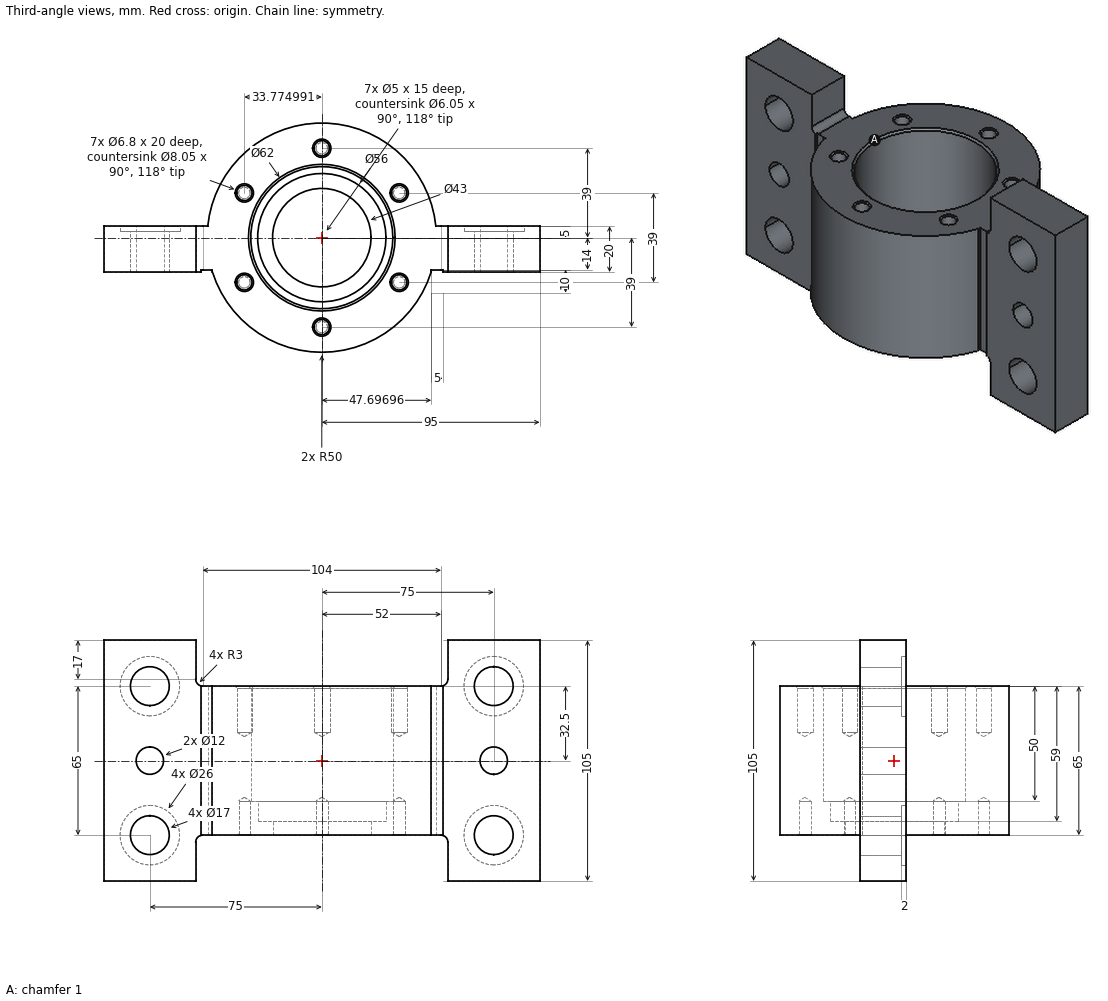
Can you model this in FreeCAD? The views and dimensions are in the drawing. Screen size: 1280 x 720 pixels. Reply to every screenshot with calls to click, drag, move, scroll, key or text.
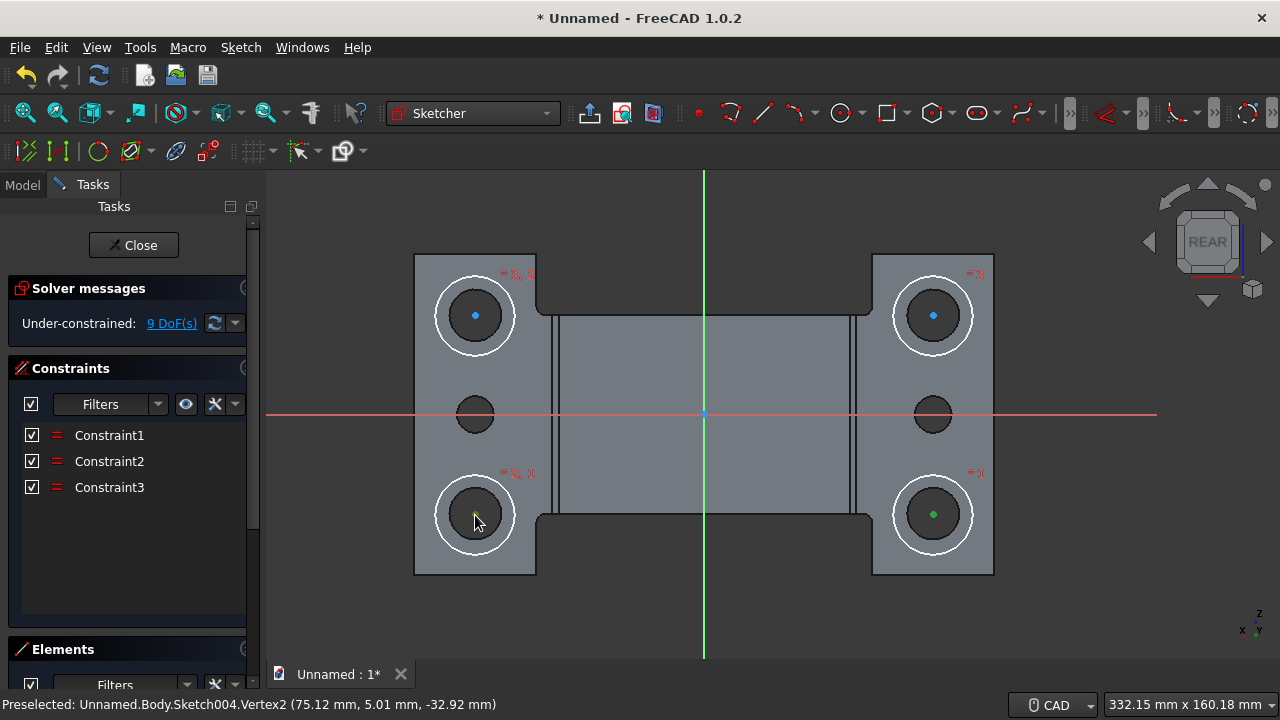
click(704, 600)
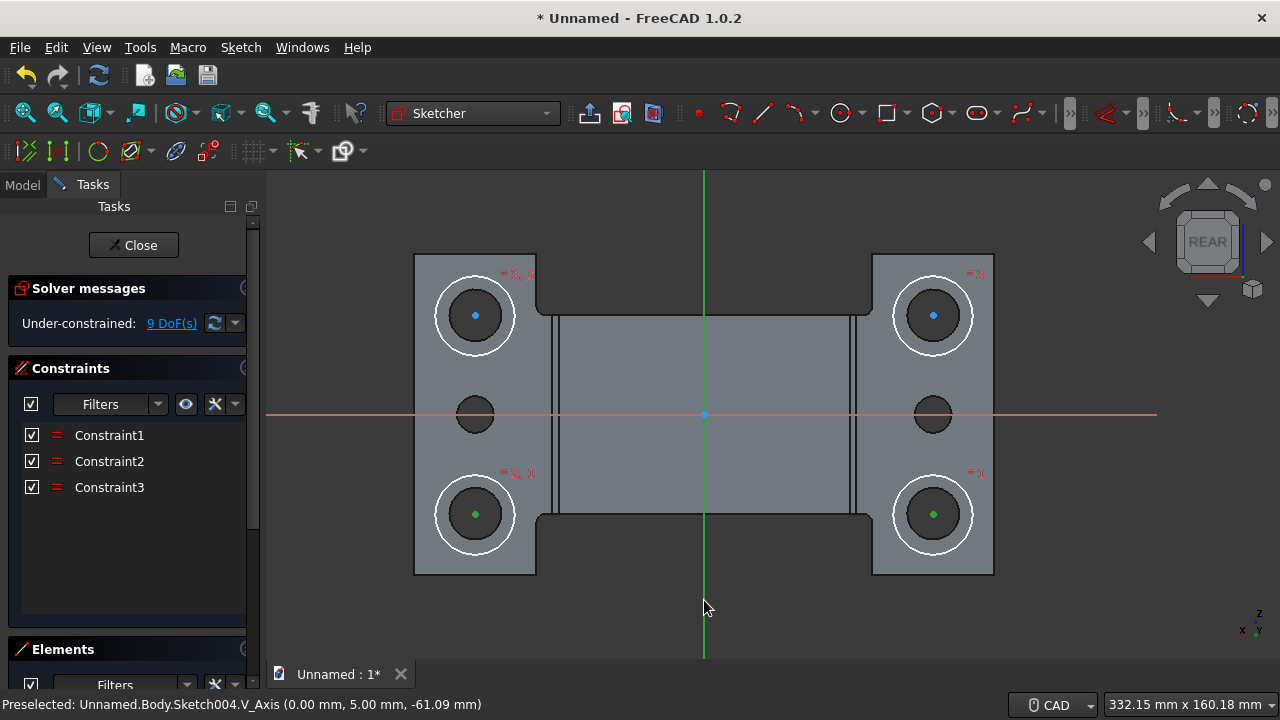
key(s)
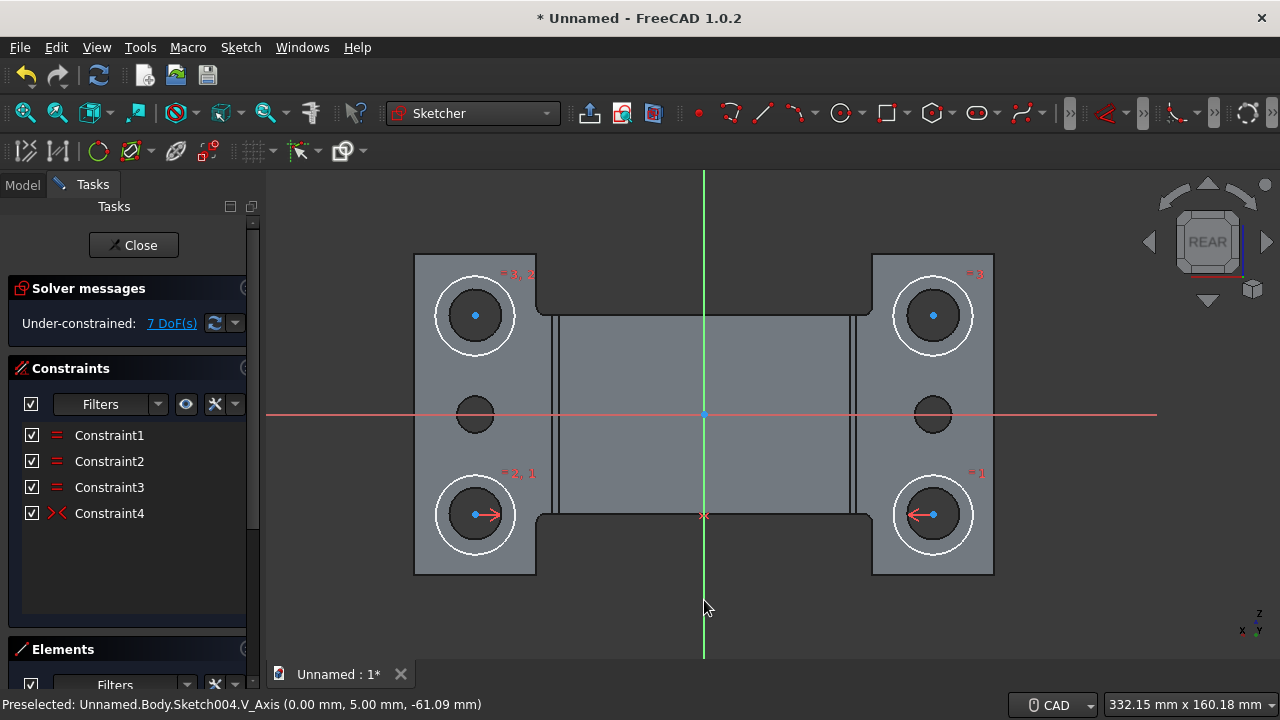
click(475, 515)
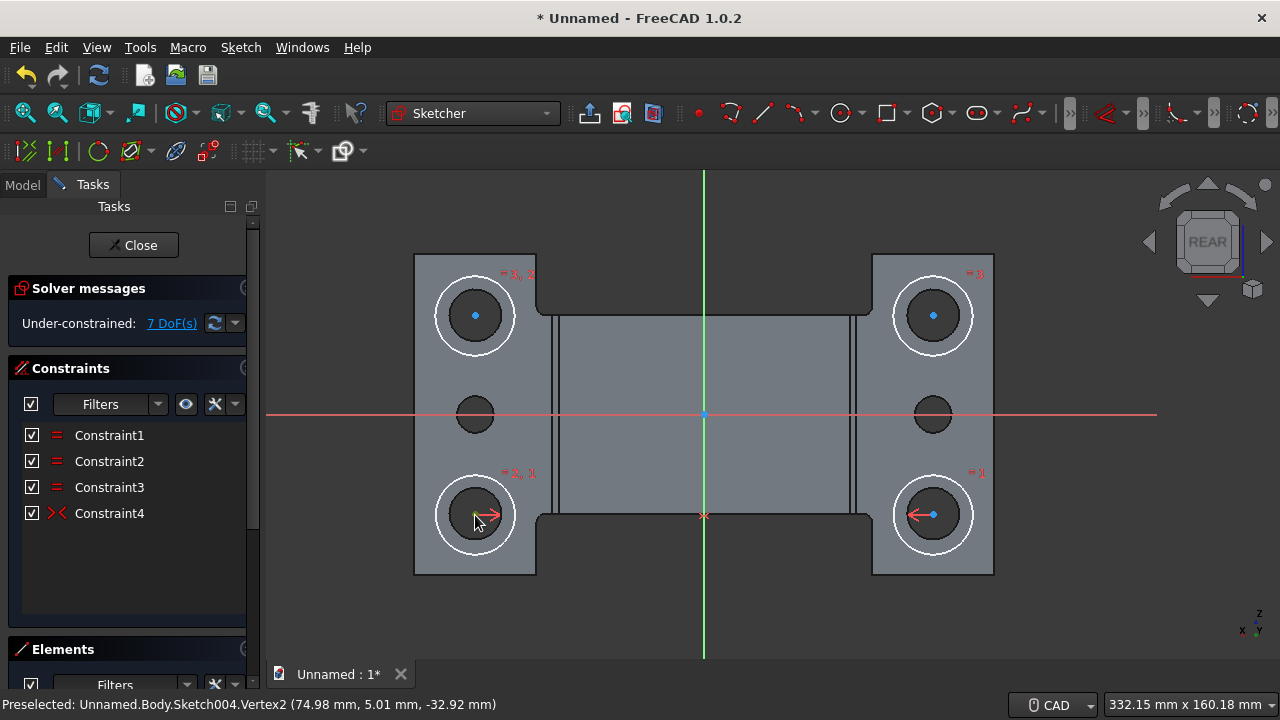
click(475, 316)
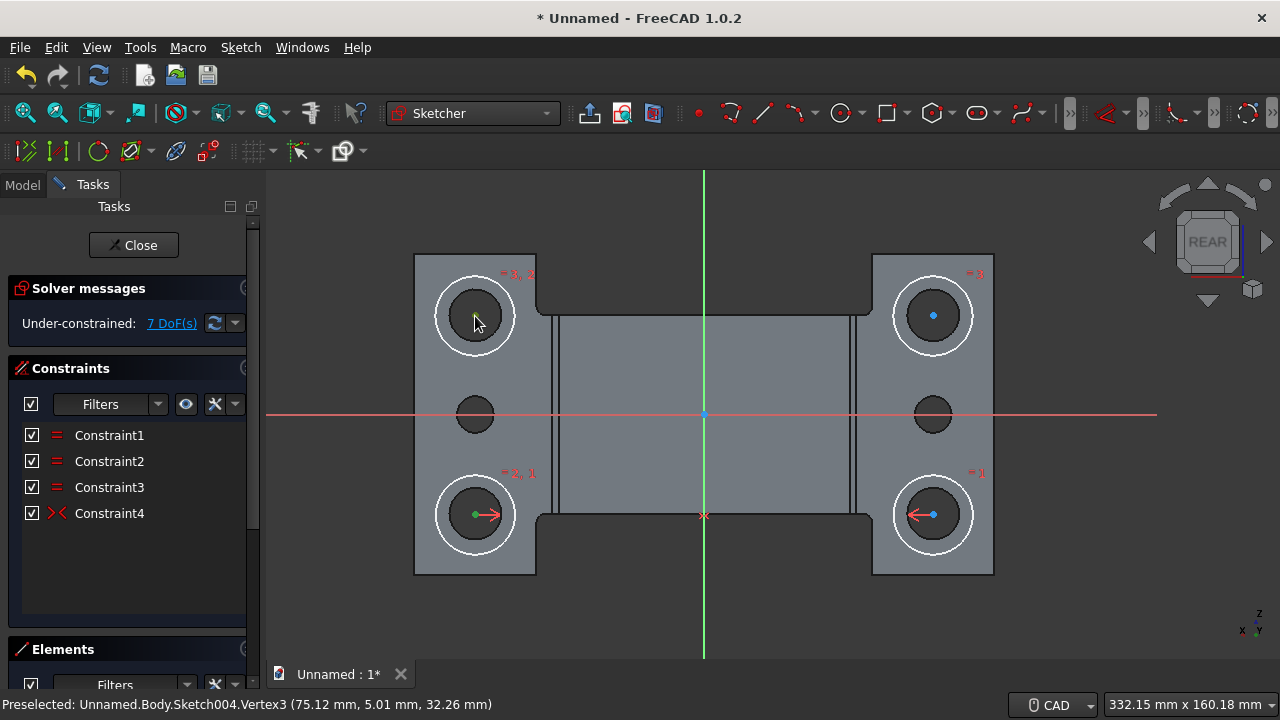
click(353, 414)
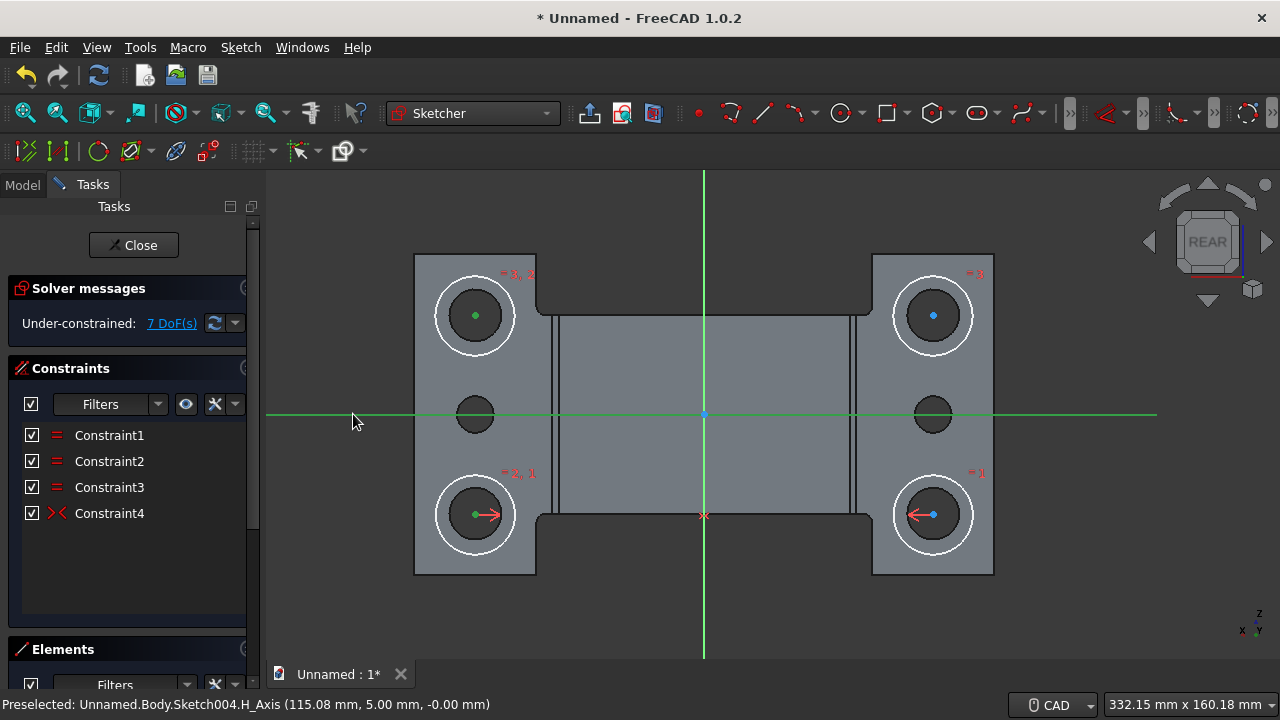
key(s)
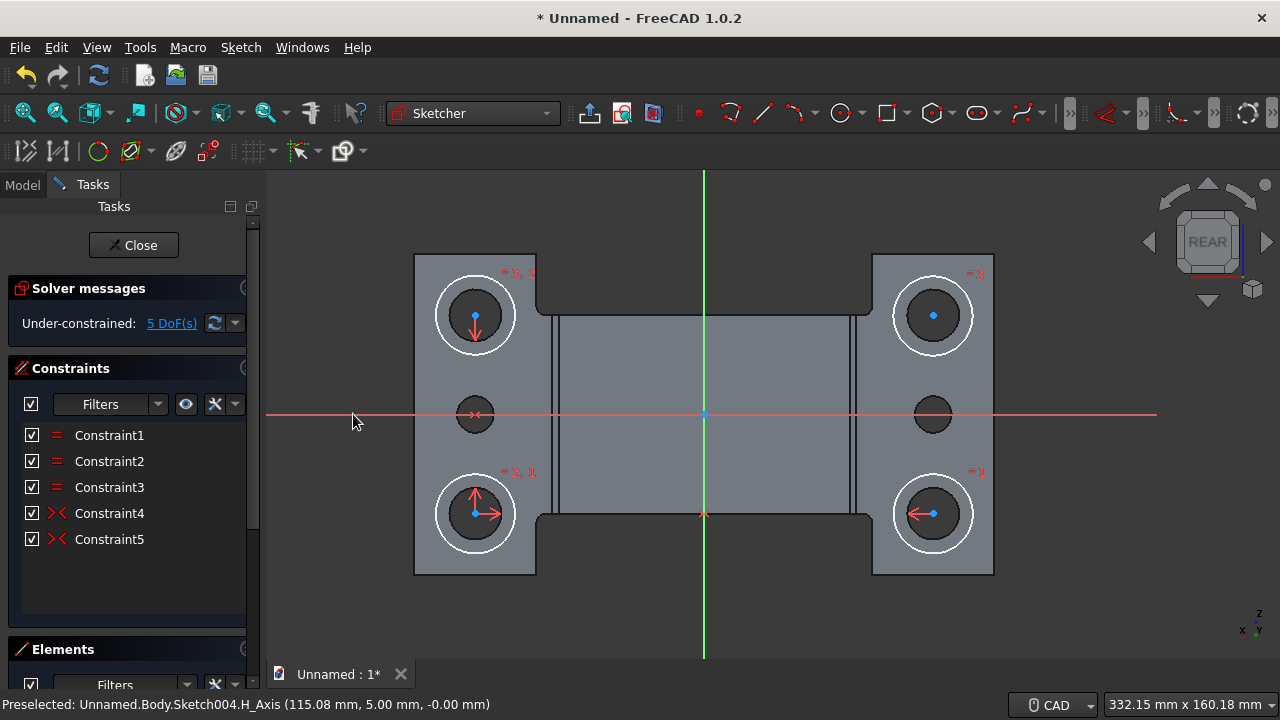
click(933, 514)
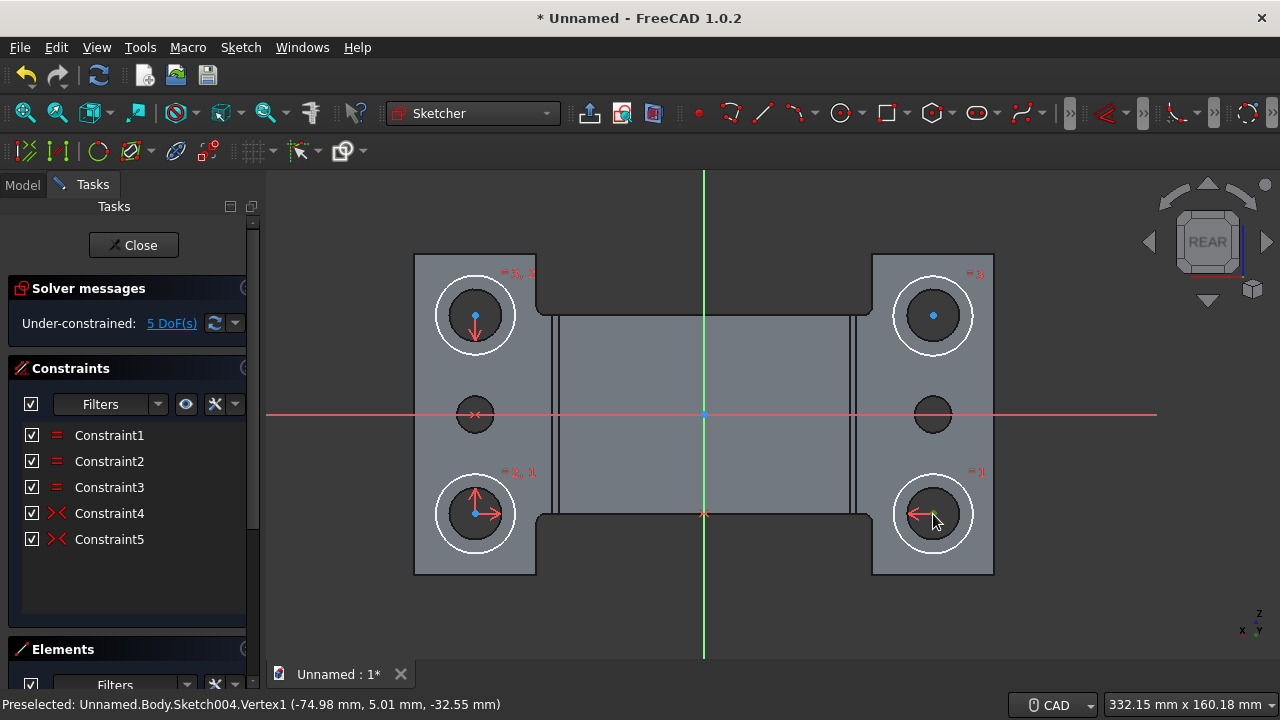
click(933, 316)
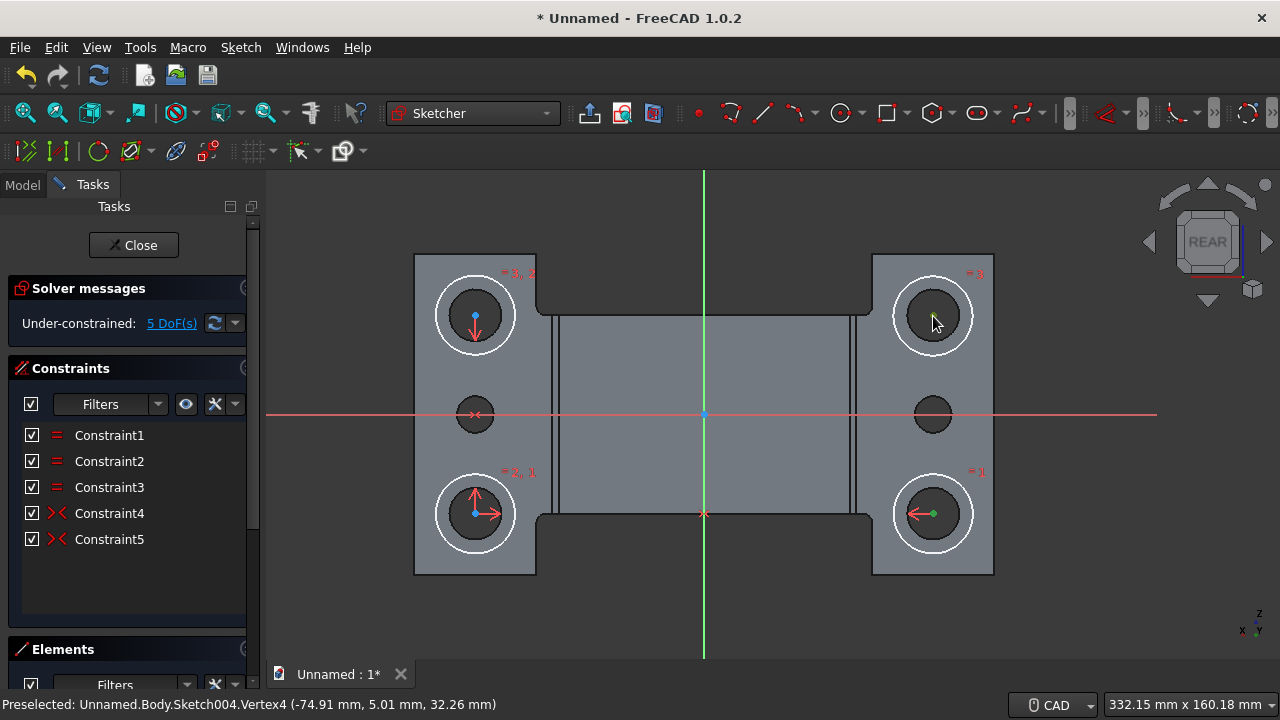
click(353, 414)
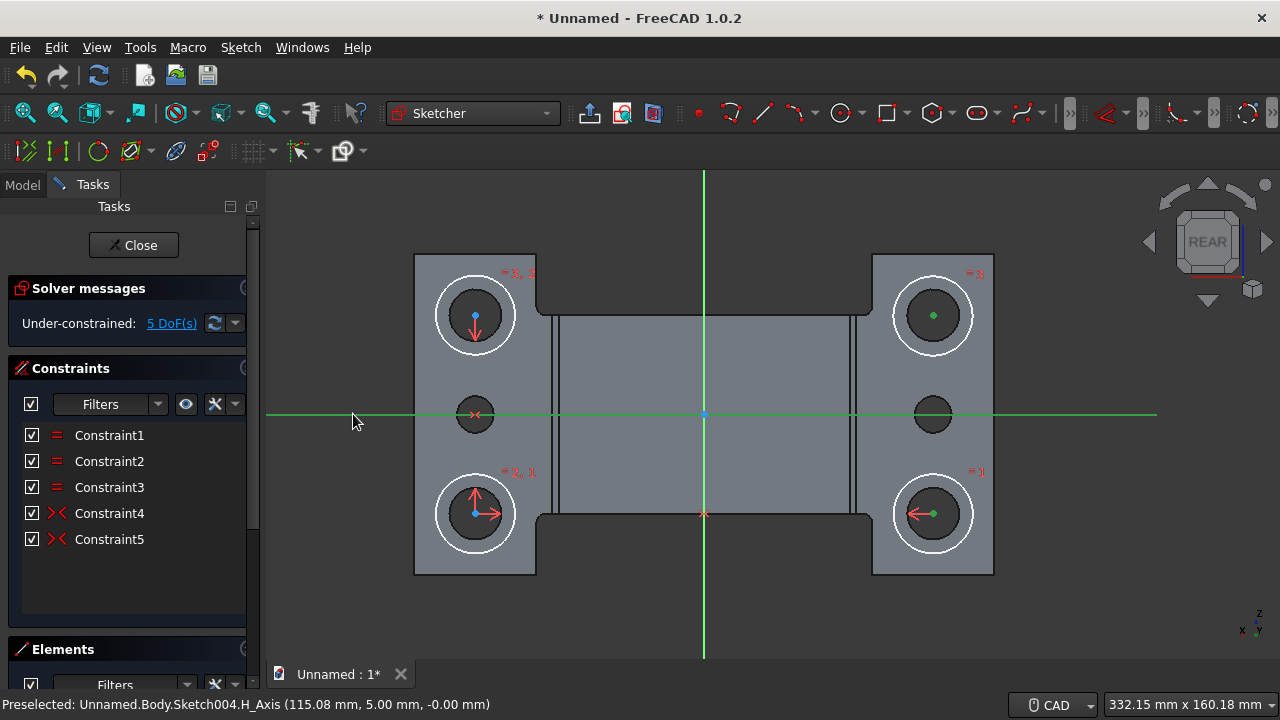
key(s)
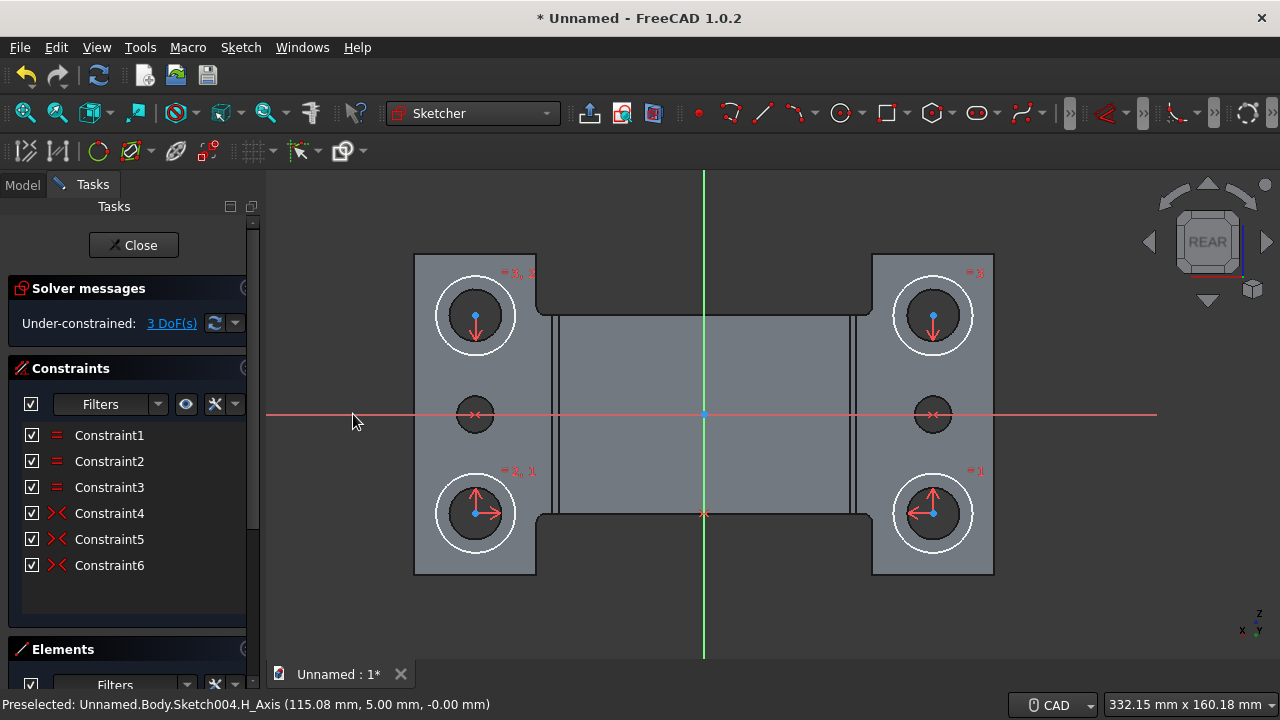
click(1106, 114)